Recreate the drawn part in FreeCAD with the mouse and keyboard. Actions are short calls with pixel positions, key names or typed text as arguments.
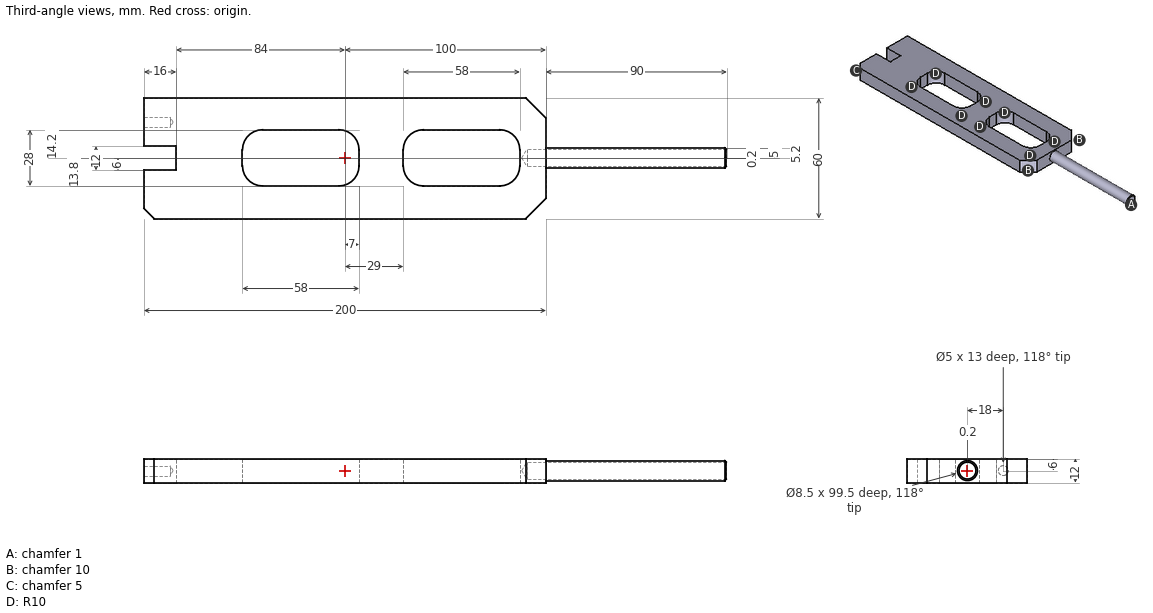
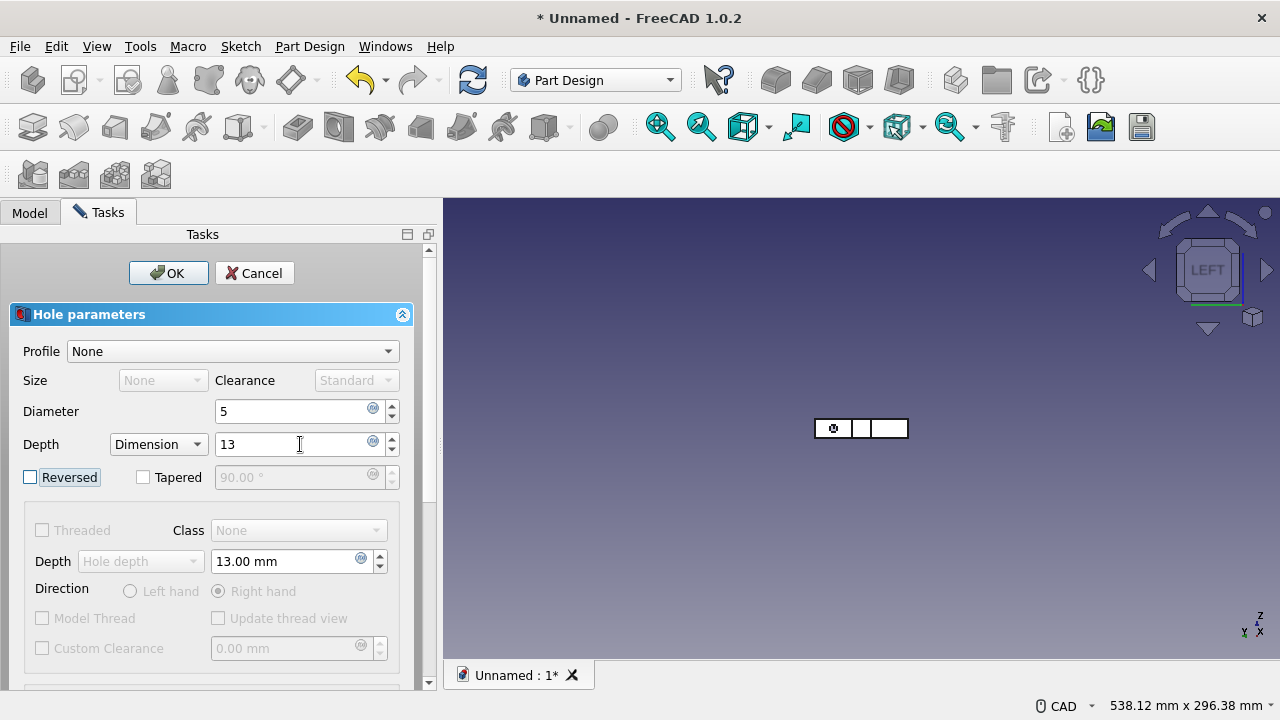
click(169, 273)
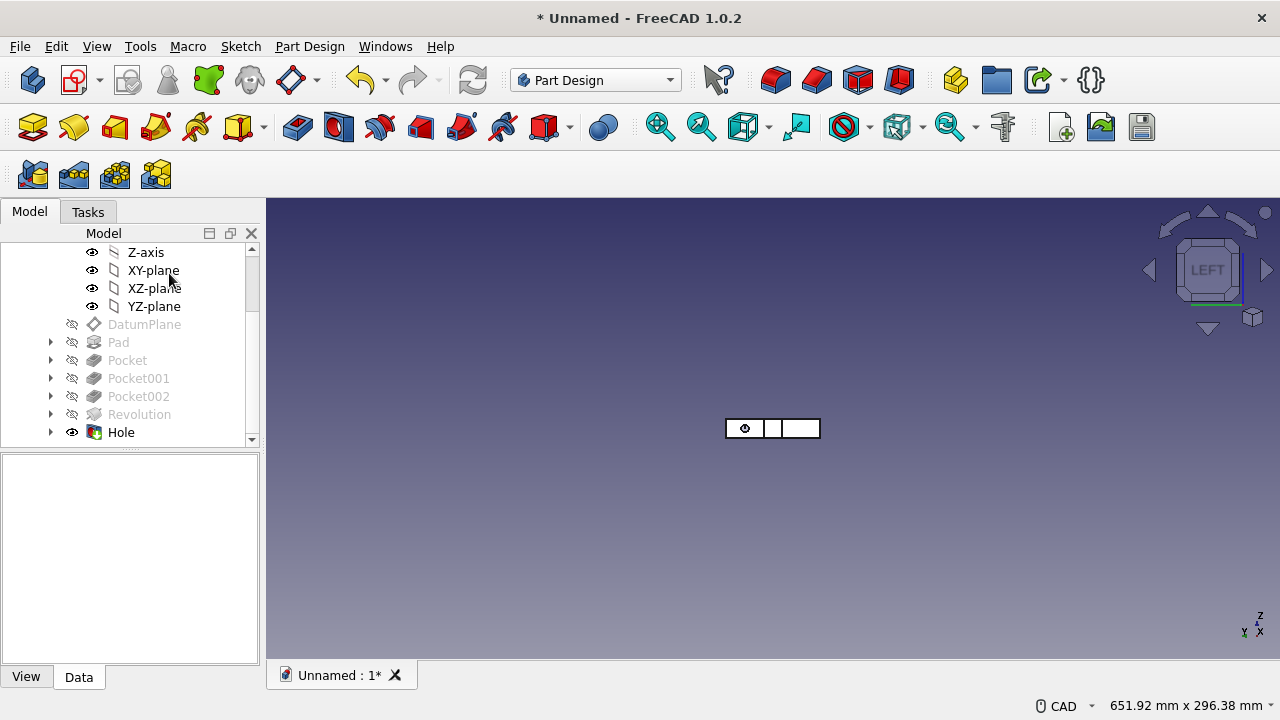
key(v)
key(f)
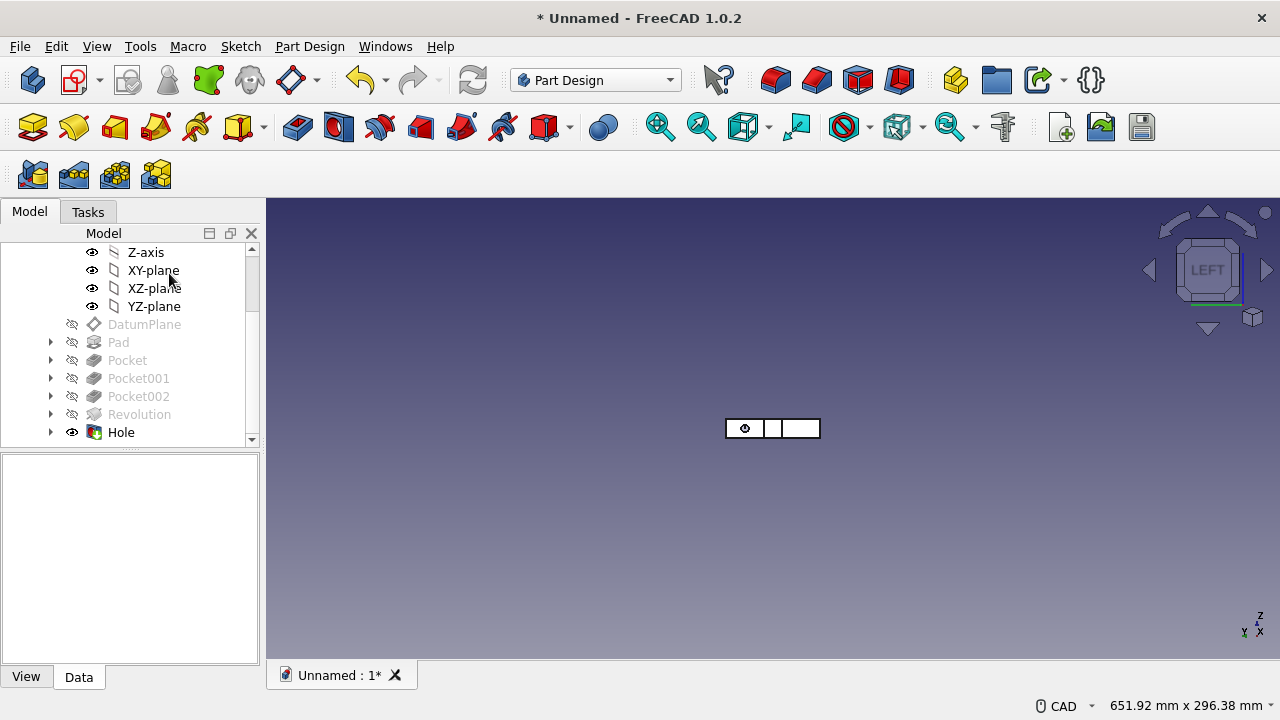
key(0)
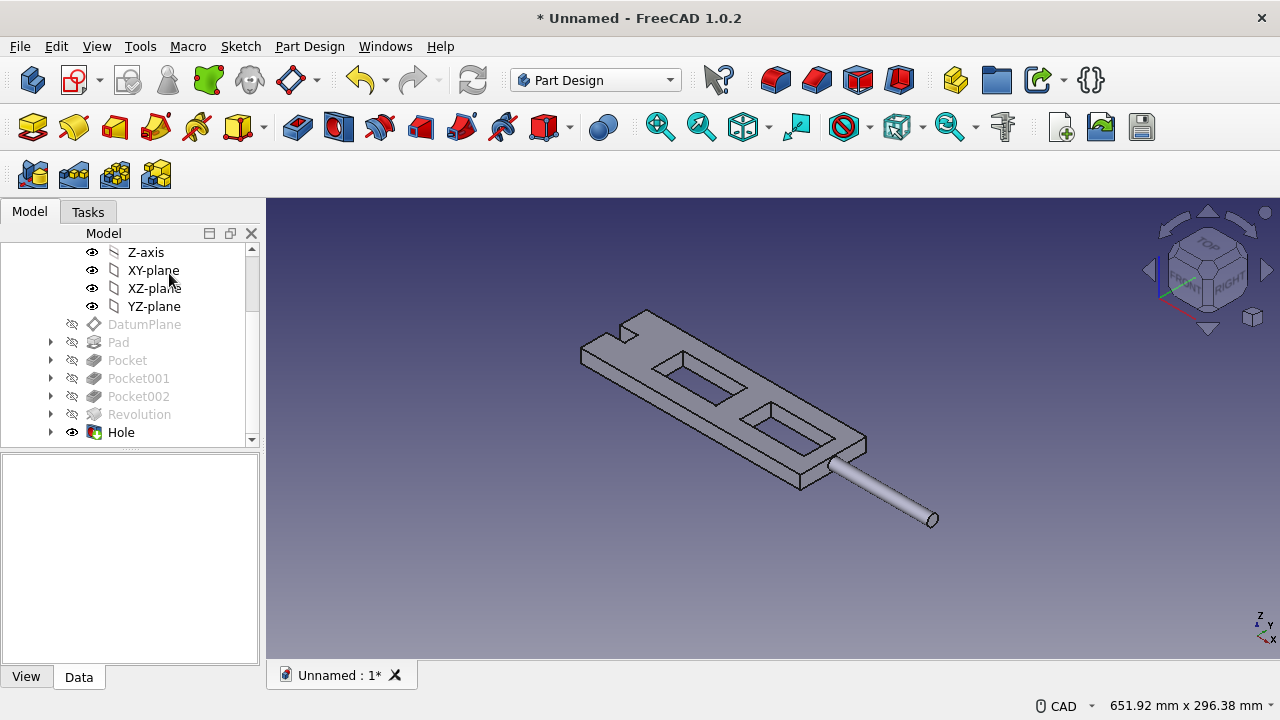
click(927, 523)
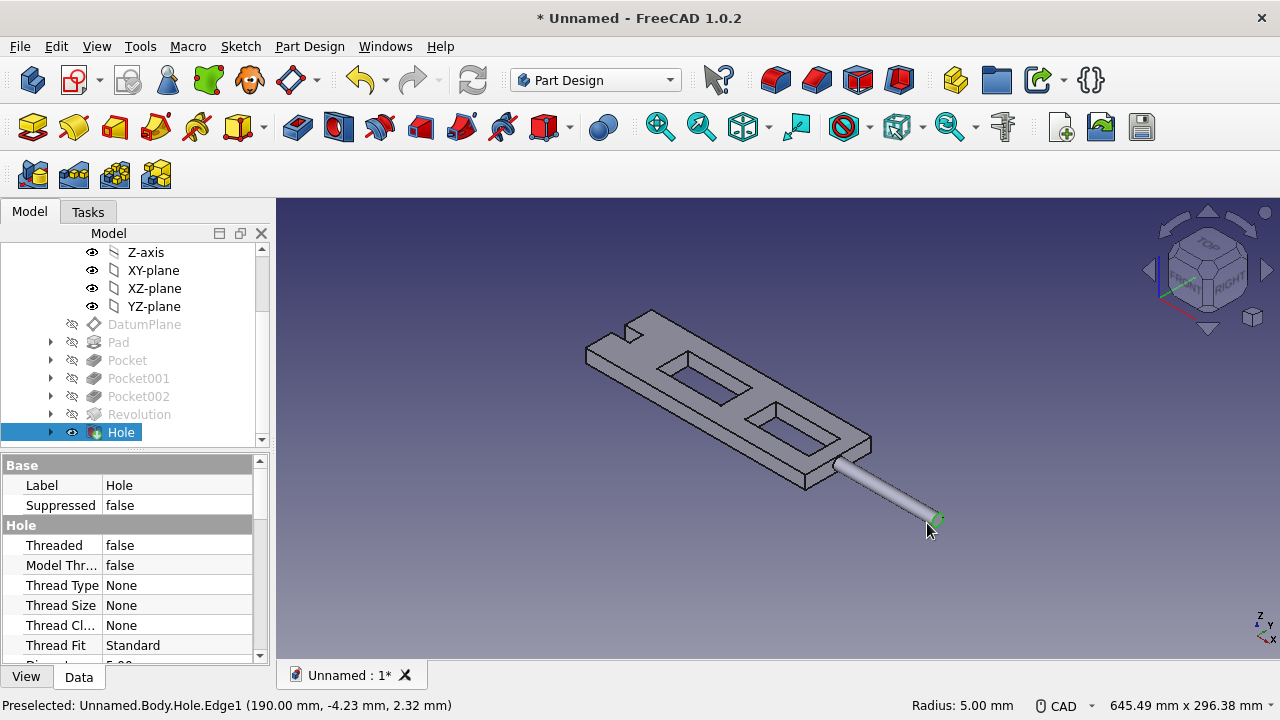
click(817, 80)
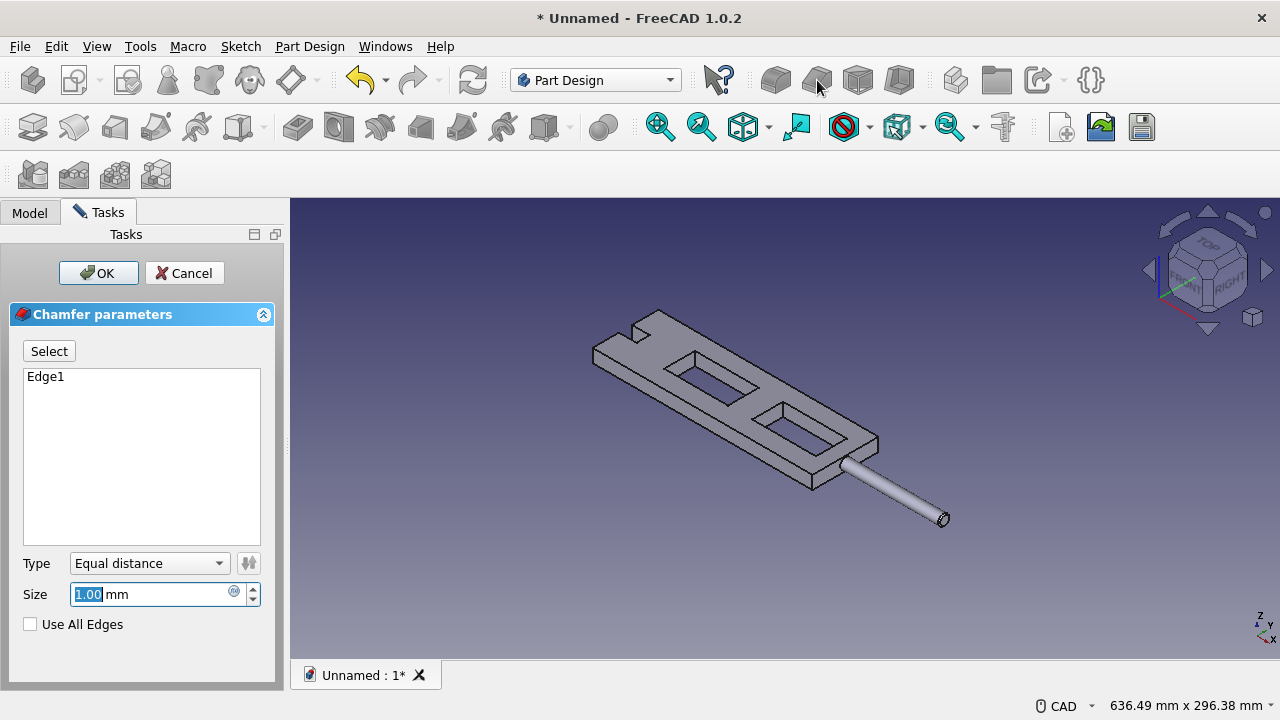
text(1)
key(Tab)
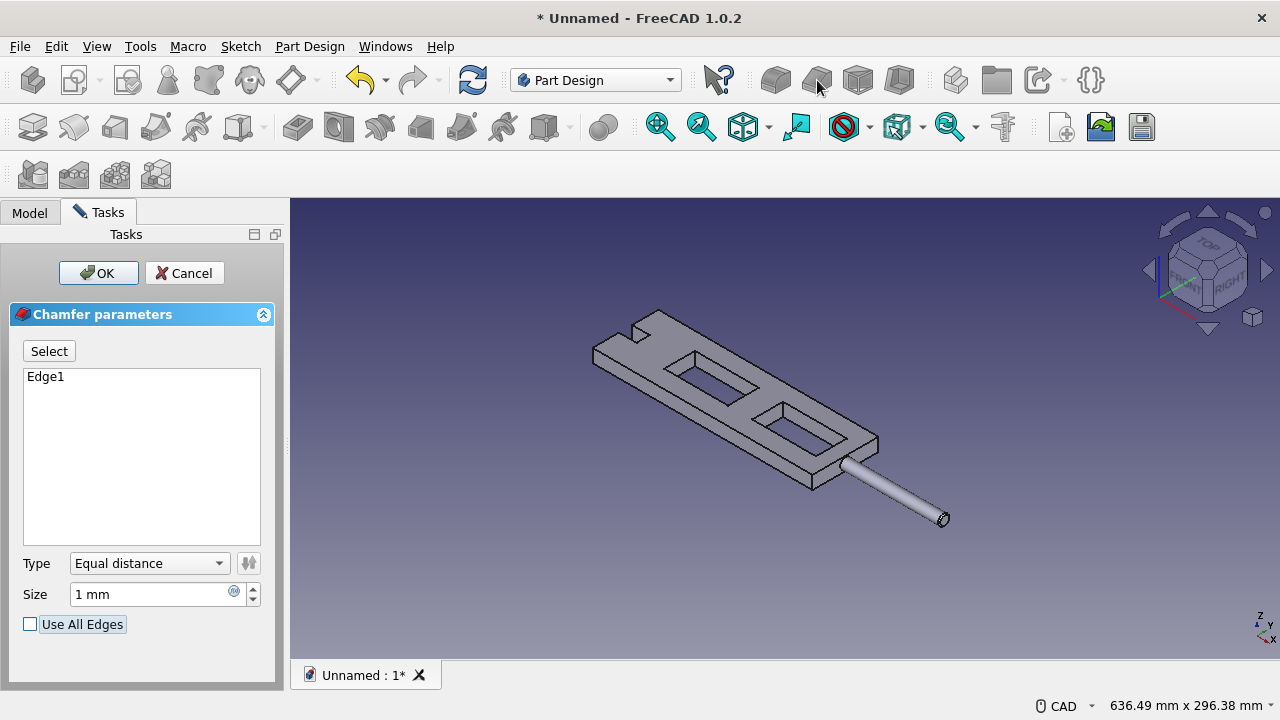
click(99, 273)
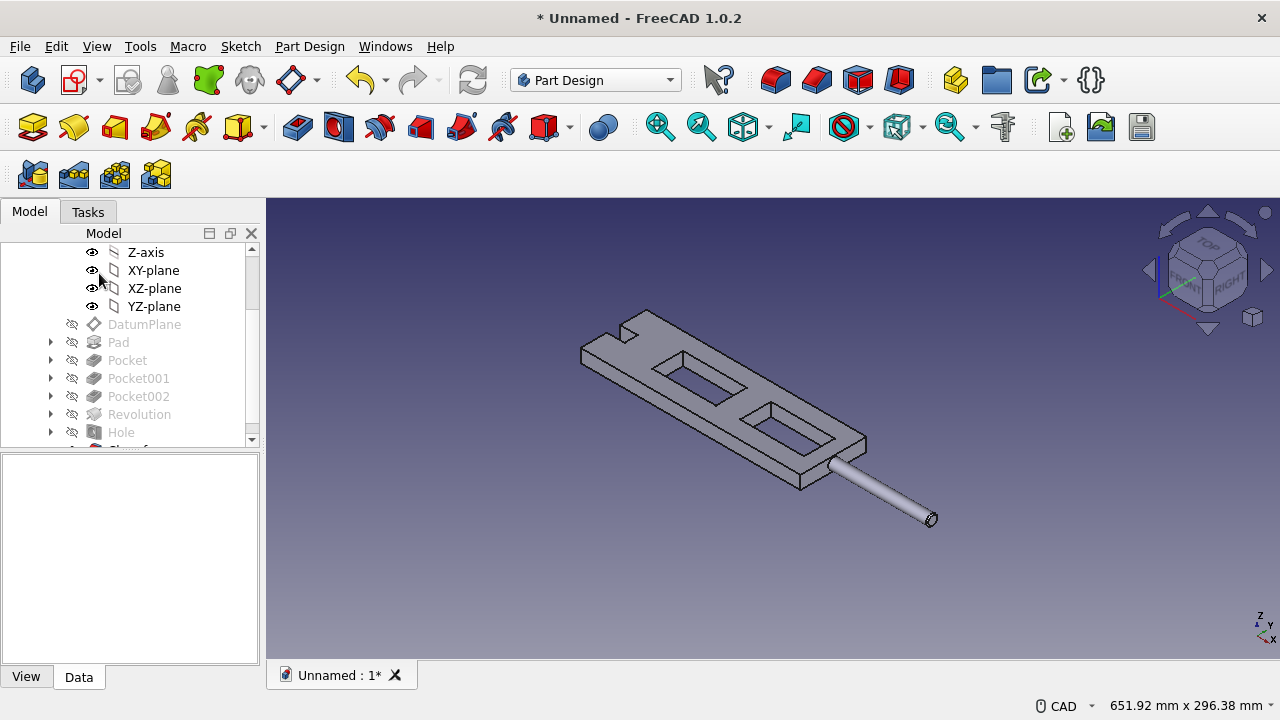
click(800, 481)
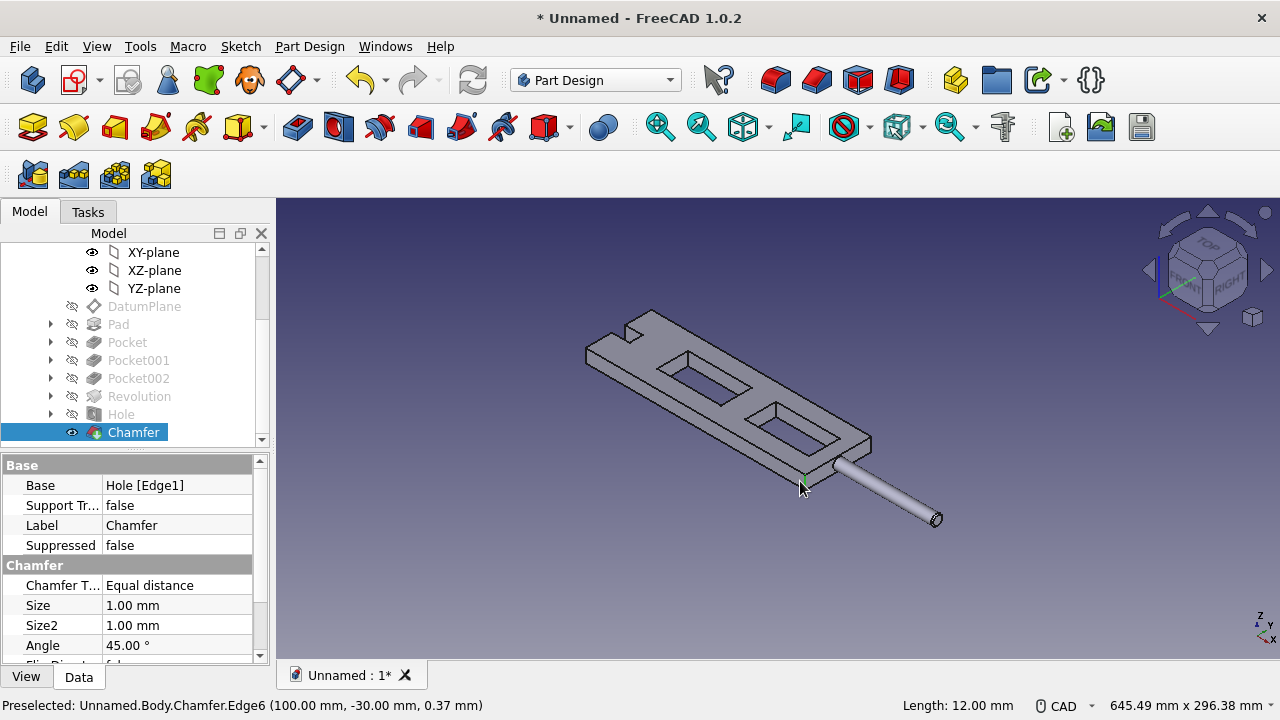
scroll(871, 443, up, 4)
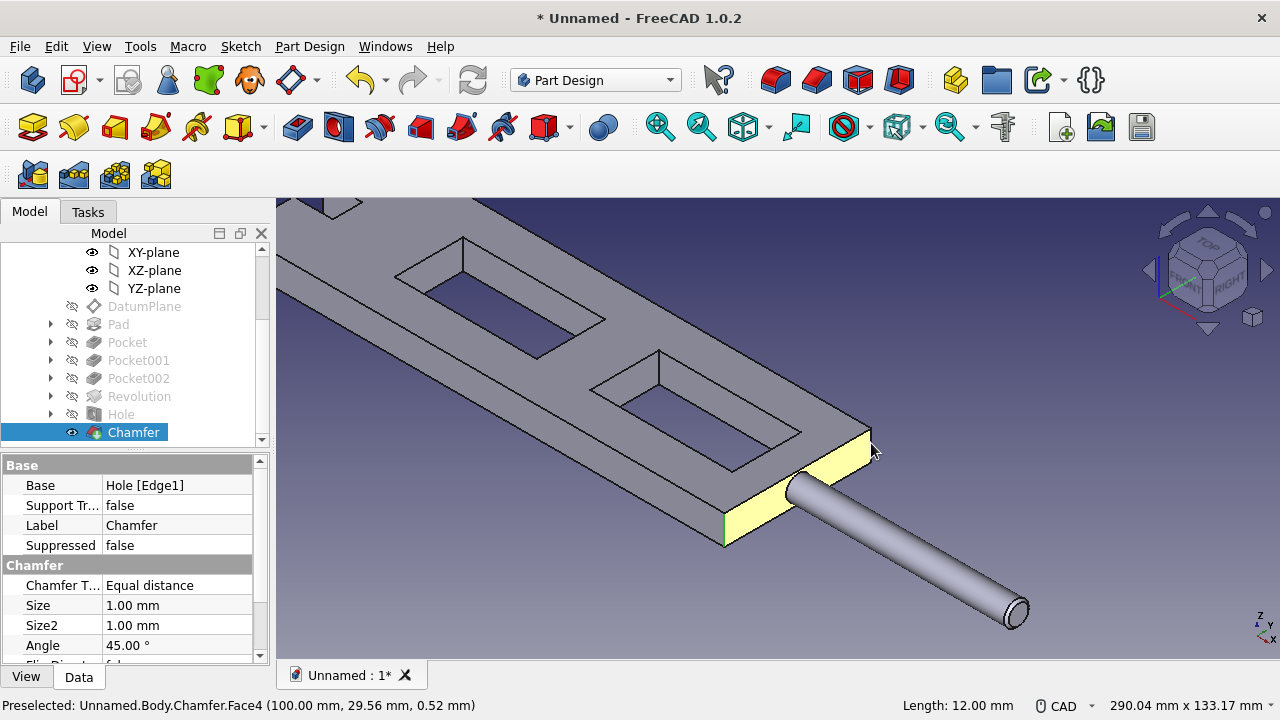
key(v)
key(f)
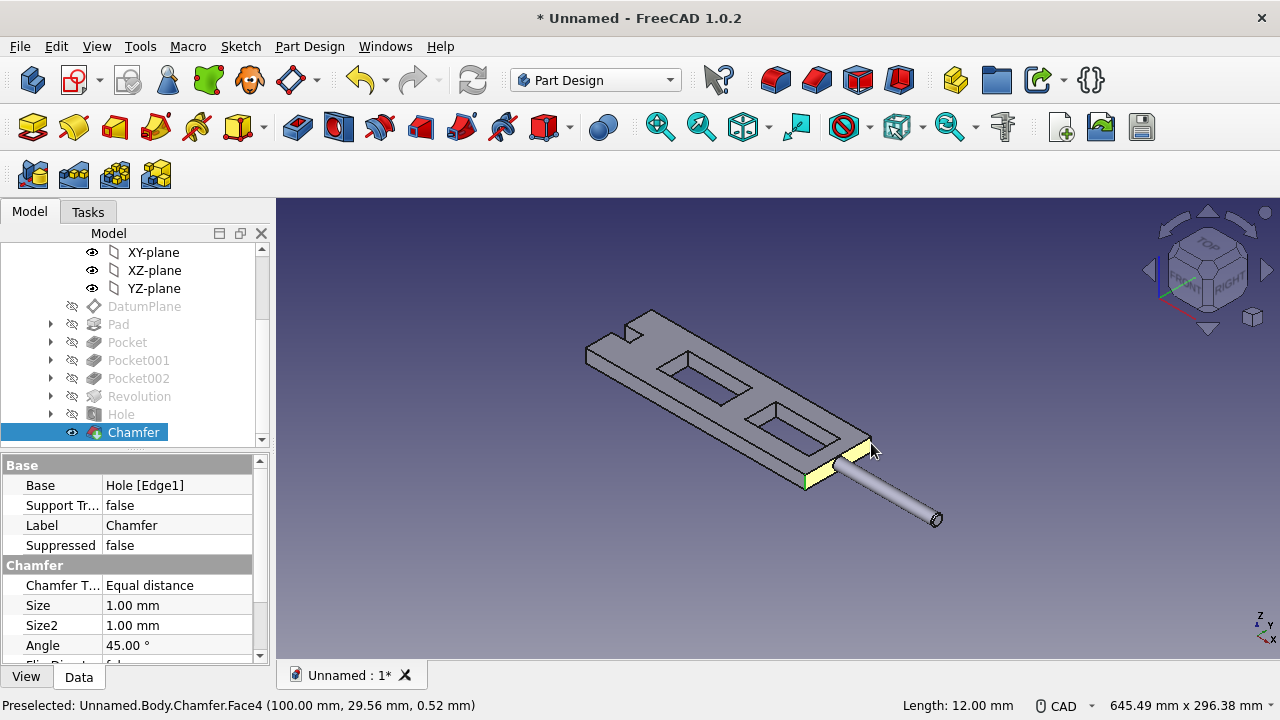
key(2)